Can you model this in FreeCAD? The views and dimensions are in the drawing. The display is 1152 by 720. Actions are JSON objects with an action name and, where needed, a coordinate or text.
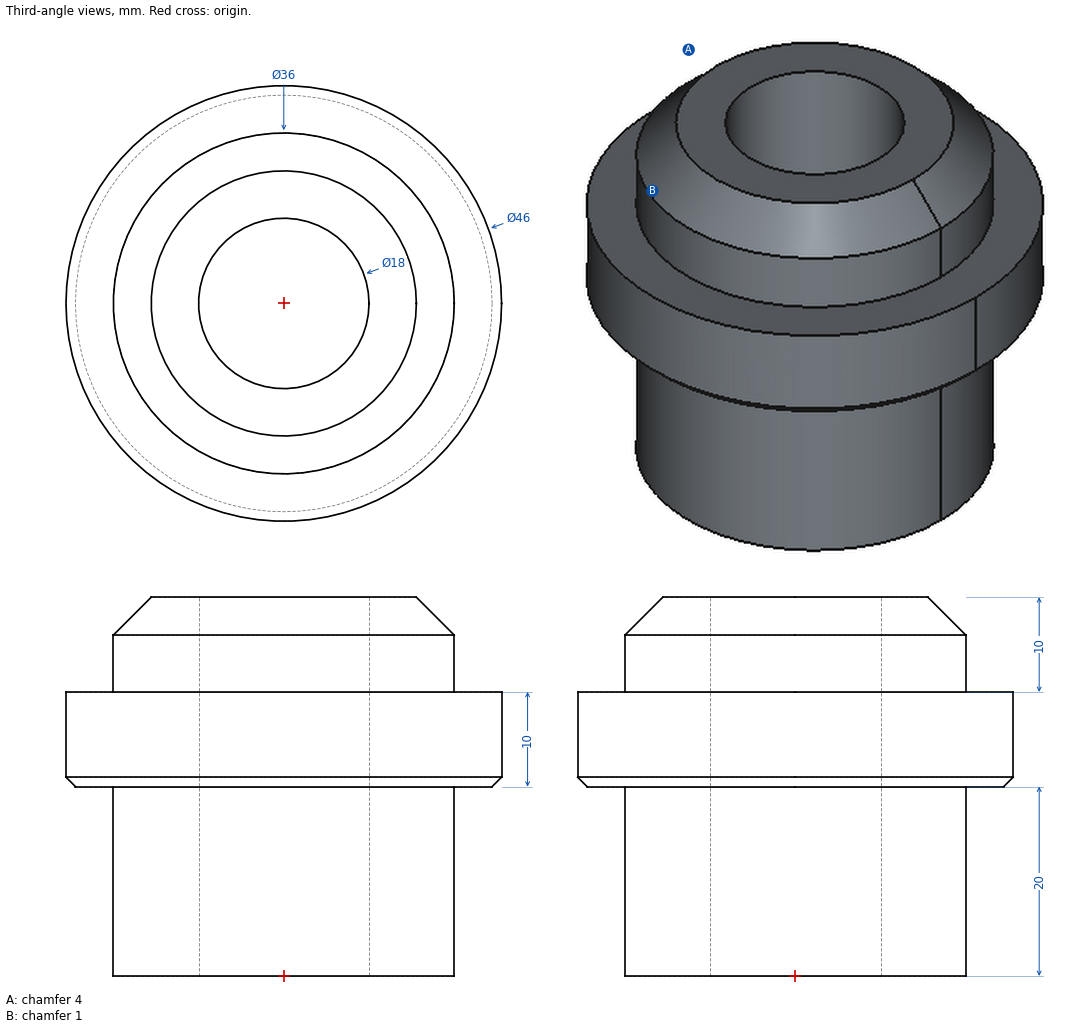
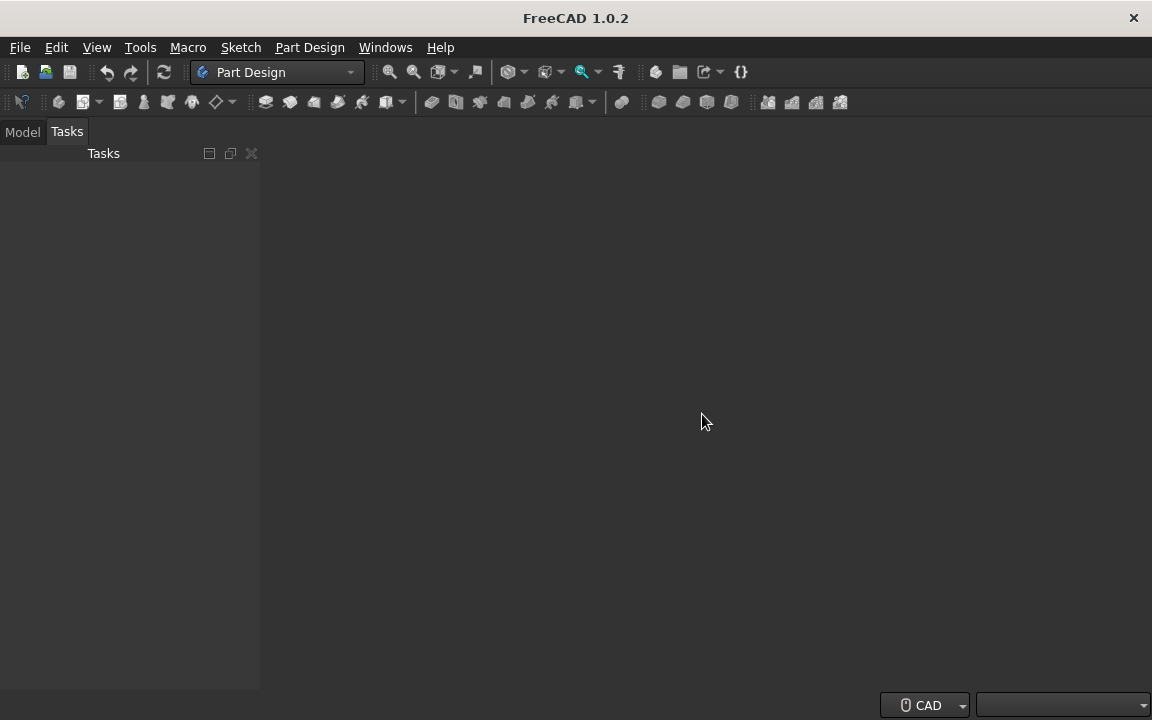
{"action": "left_click", "coordinate": [22, 72]}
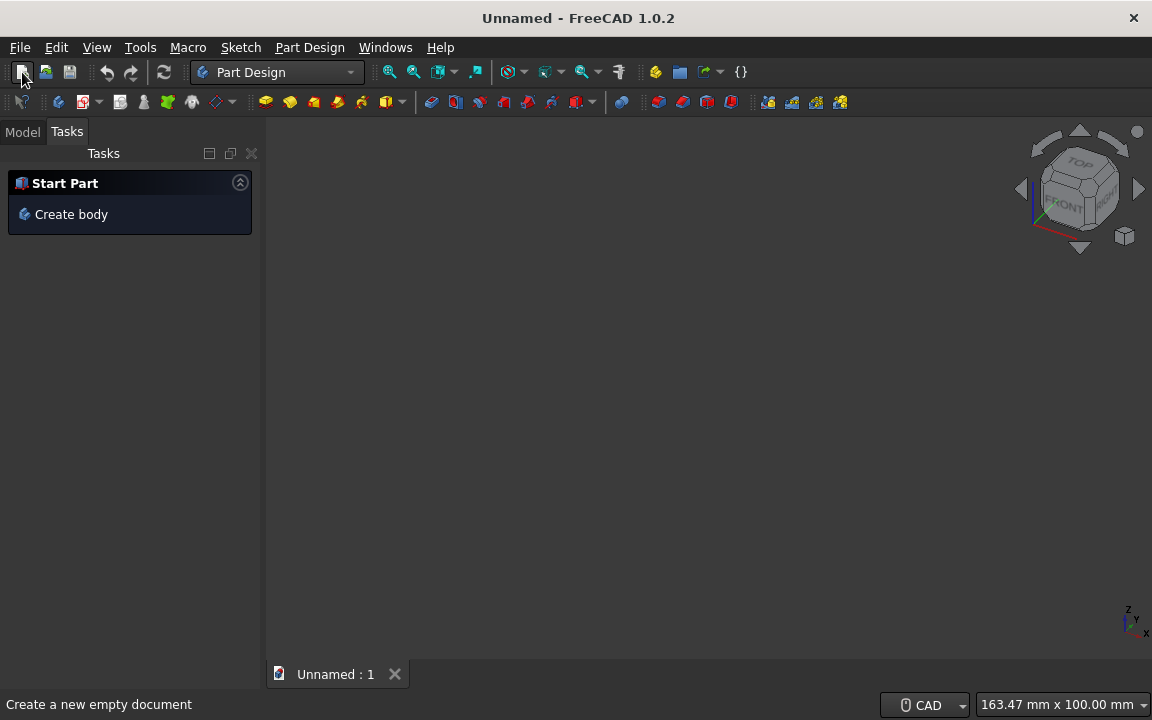
{"action": "left_click", "coordinate": [84, 102]}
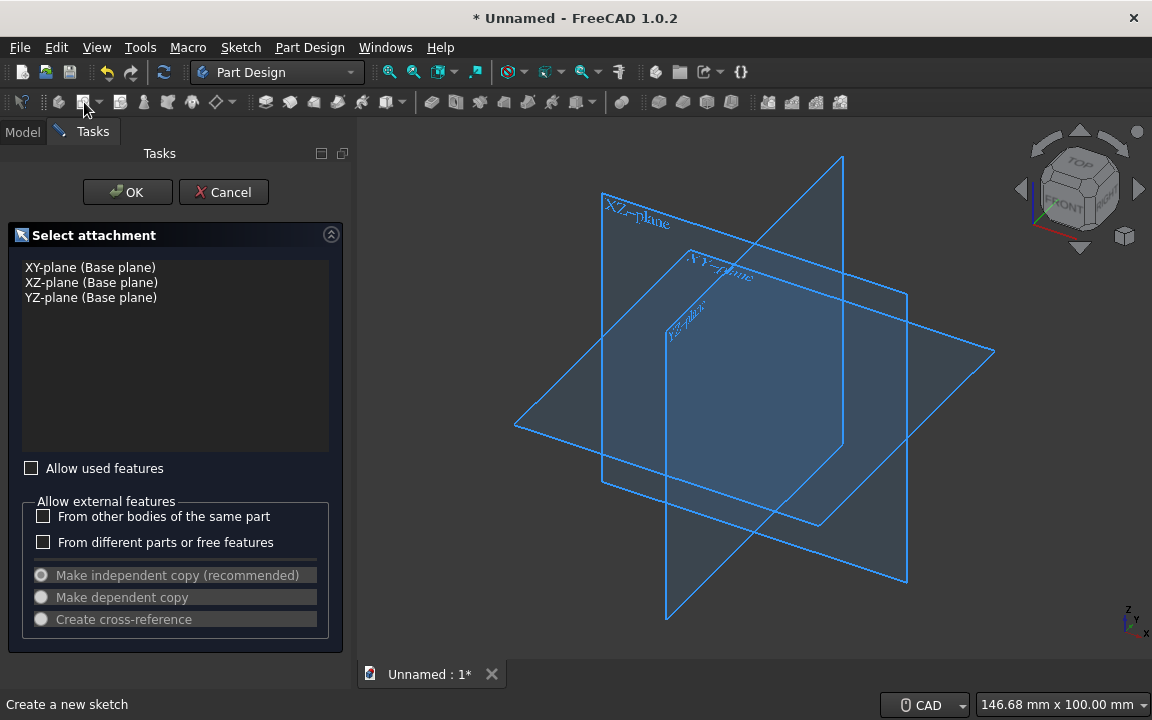
{"action": "left_click", "coordinate": [82, 268]}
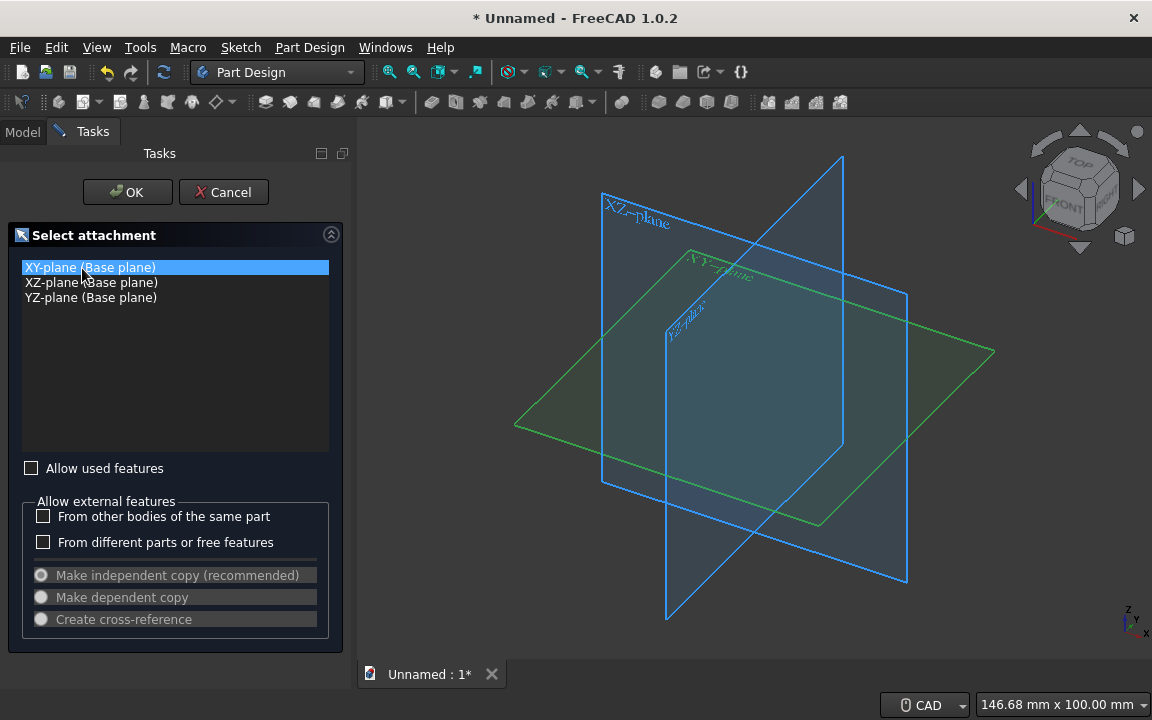
{"action": "left_click", "coordinate": [128, 192]}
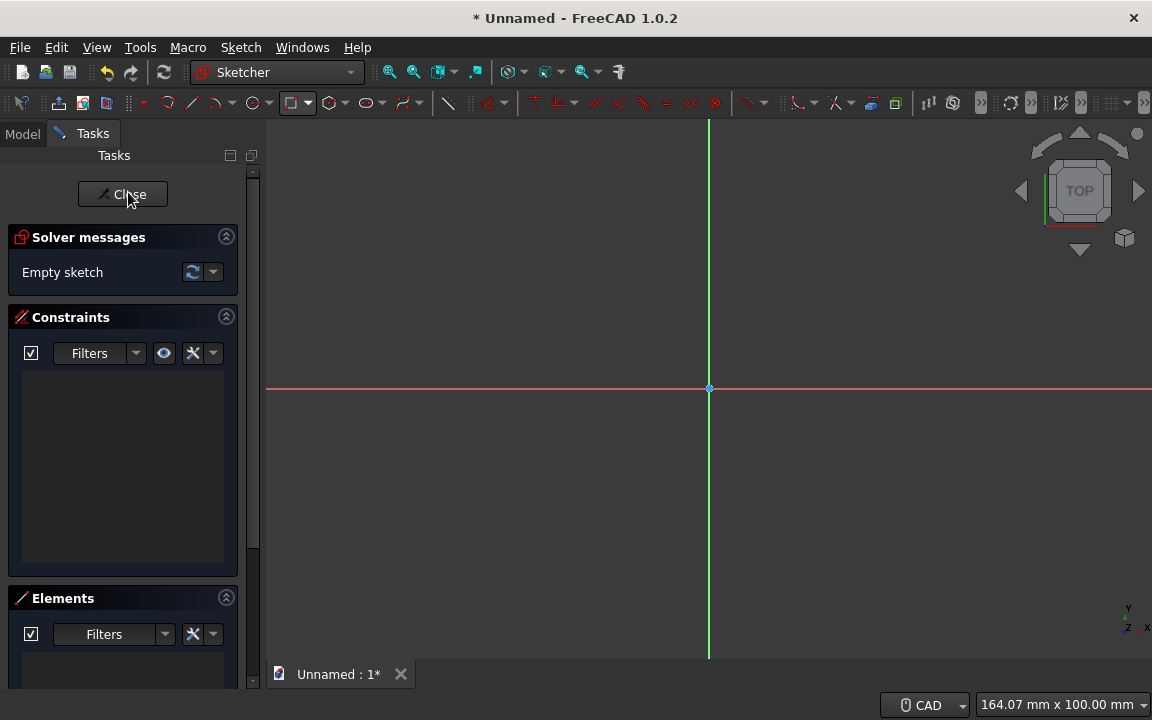
{"action": "scroll", "coordinate": [792, 389], "scroll_direction": "up", "scroll_amount": 3}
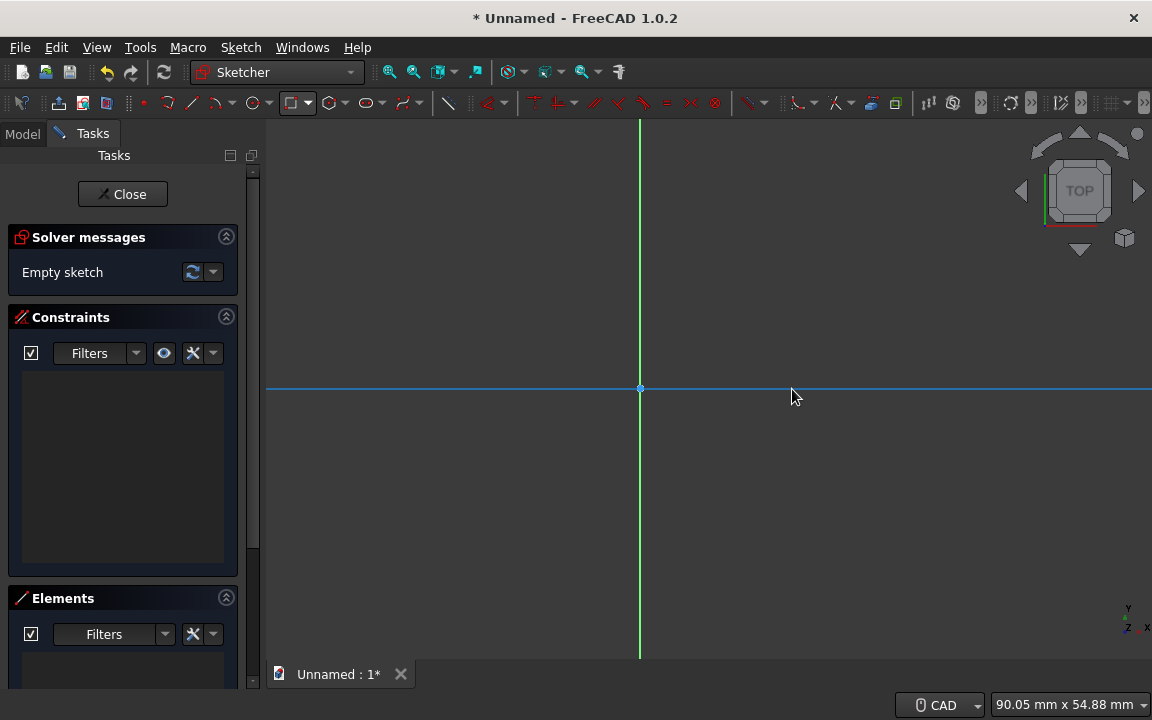
{"action": "key", "text": "g c"}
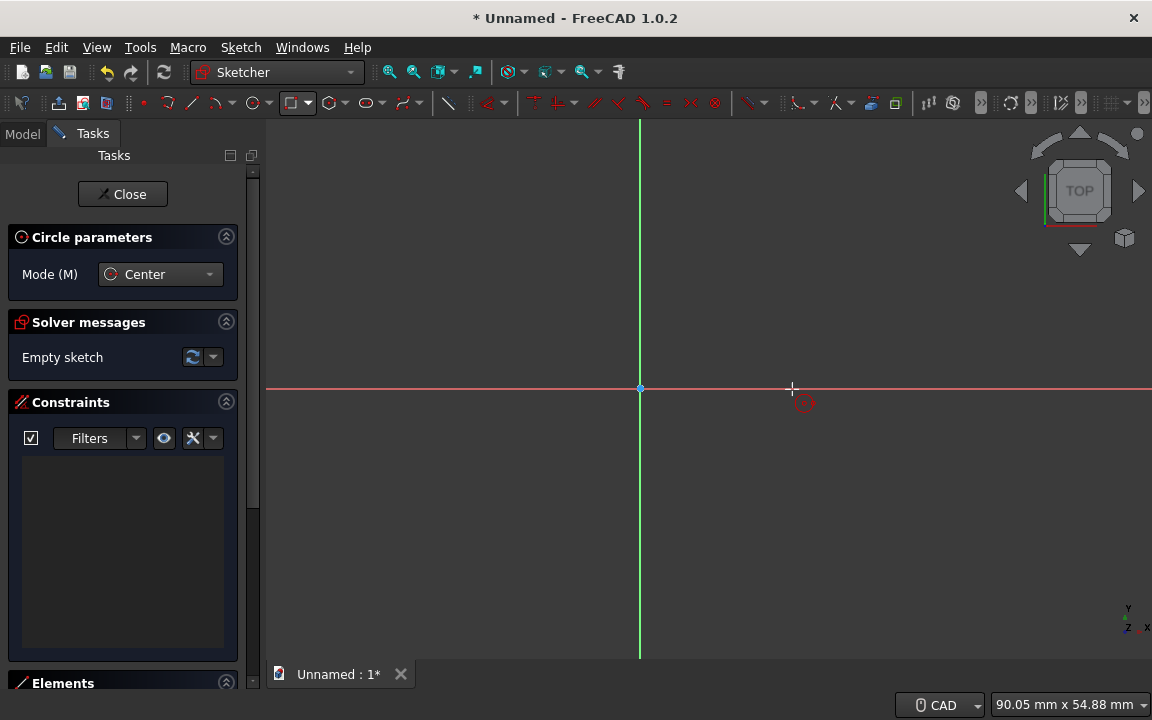
{"action": "left_click", "coordinate": [640, 389]}
{"action": "left_click", "coordinate": [766, 263]}
{"action": "key", "text": "Escape"}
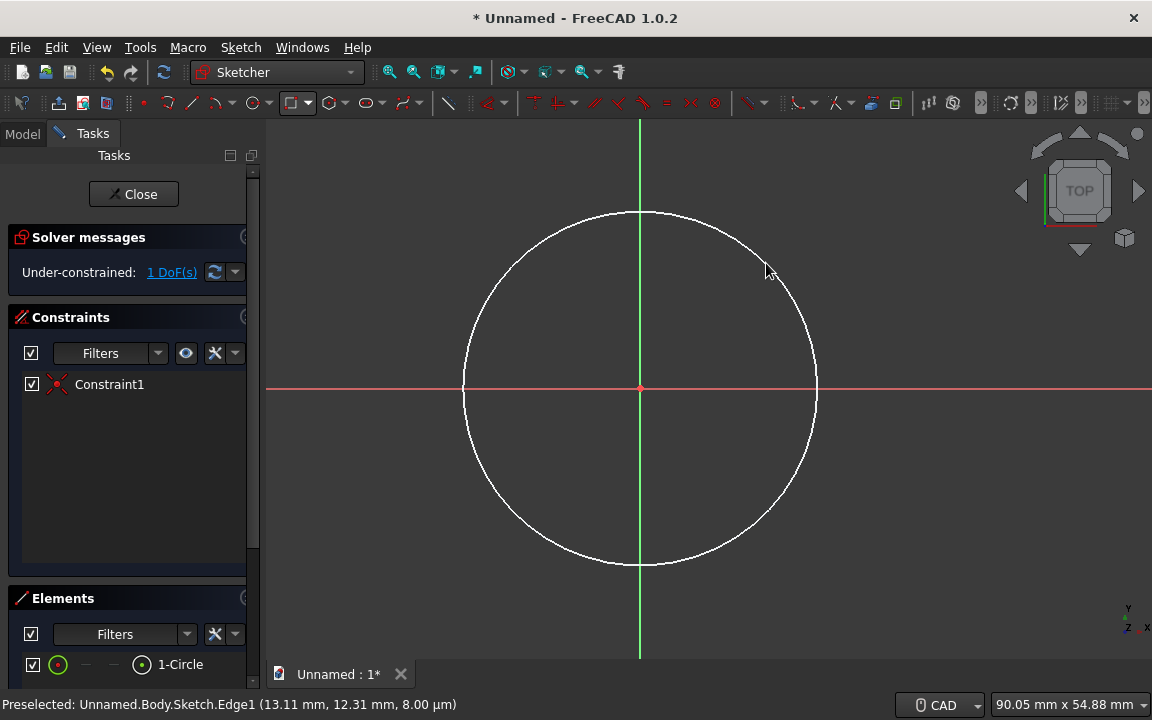
{"action": "left_click", "coordinate": [488, 104]}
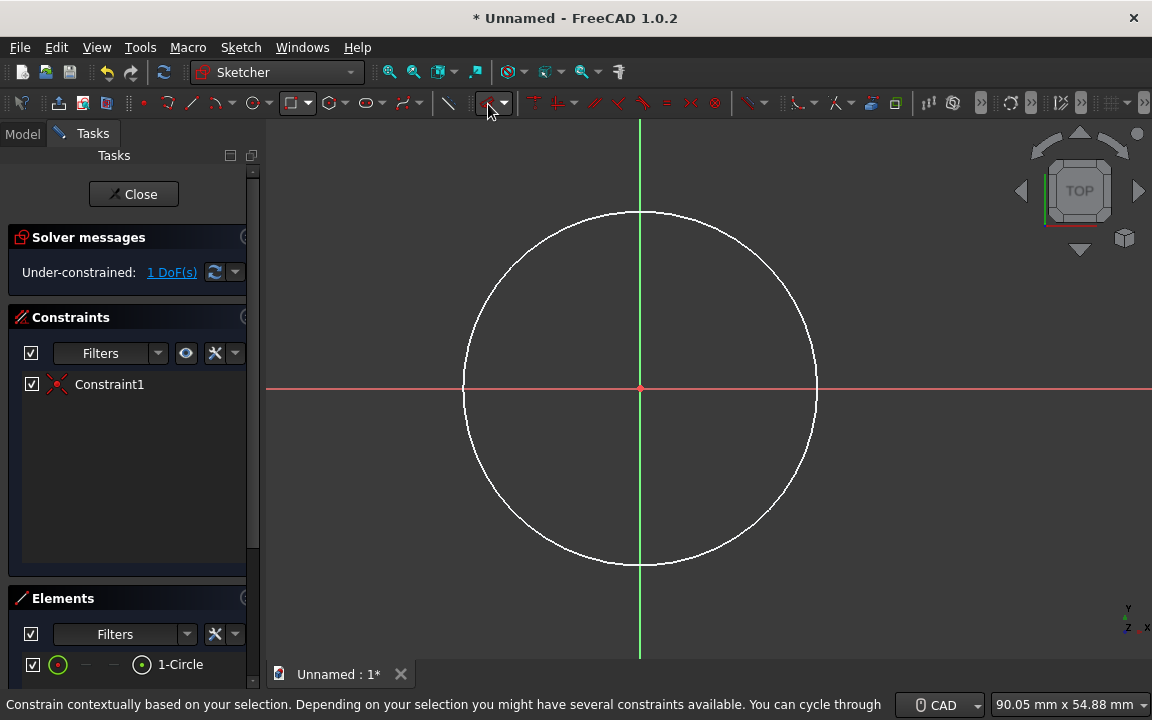
{"action": "left_click", "coordinate": [765, 263]}
{"action": "left_click", "coordinate": [788, 240]}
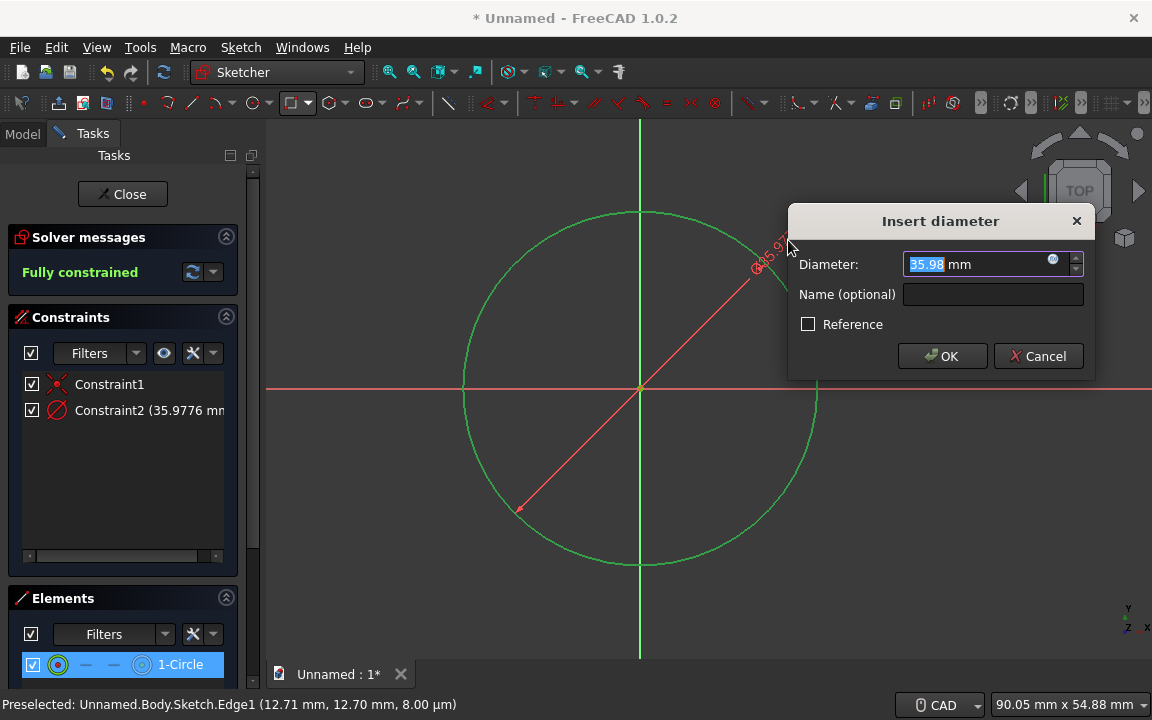
{"action": "type", "text": "36"}
{"action": "key", "text": "Return"}
{"action": "key", "text": "Escape"}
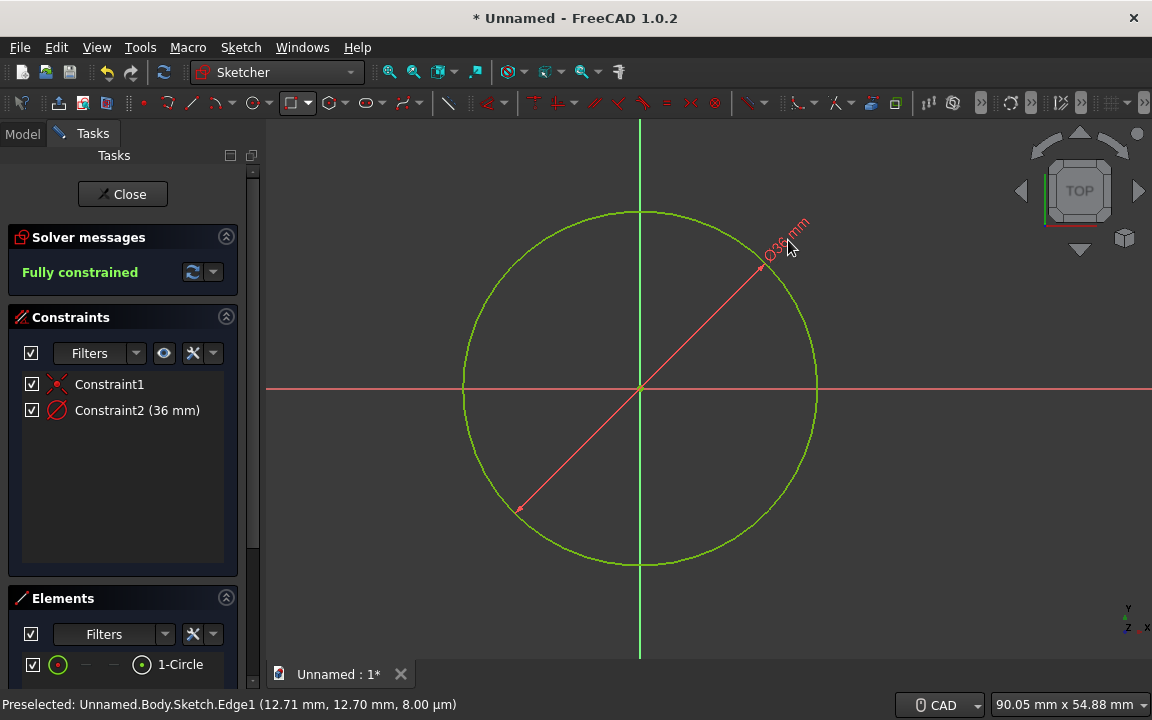
{"action": "left_click", "coordinate": [123, 194]}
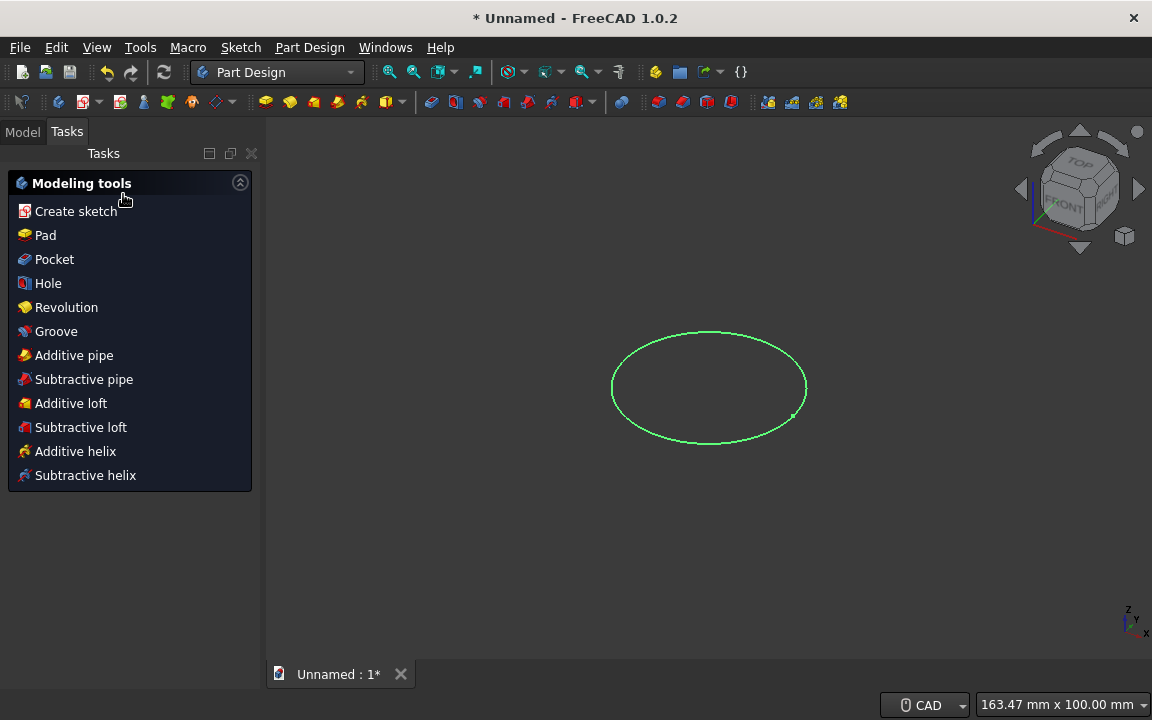
{"action": "left_click", "coordinate": [266, 102]}